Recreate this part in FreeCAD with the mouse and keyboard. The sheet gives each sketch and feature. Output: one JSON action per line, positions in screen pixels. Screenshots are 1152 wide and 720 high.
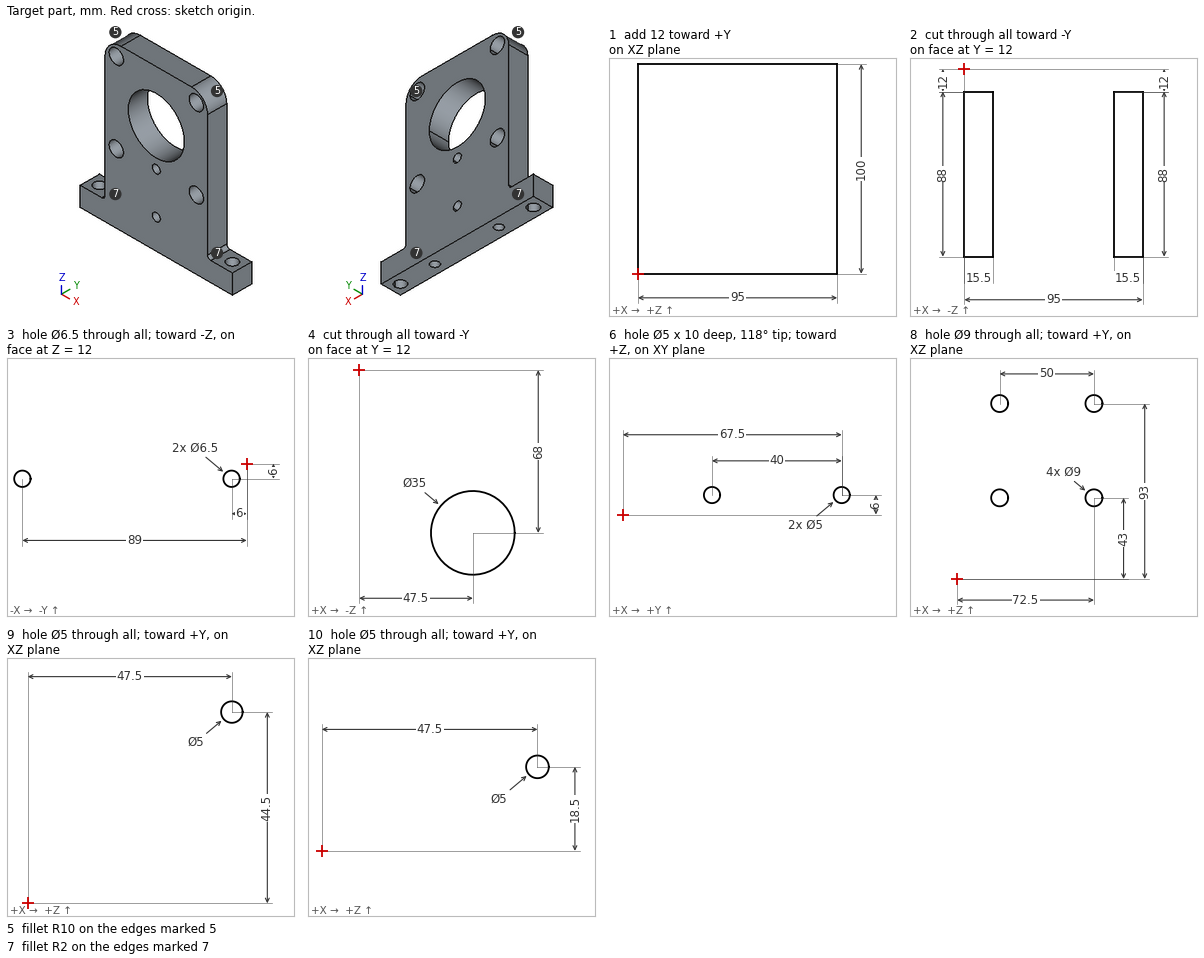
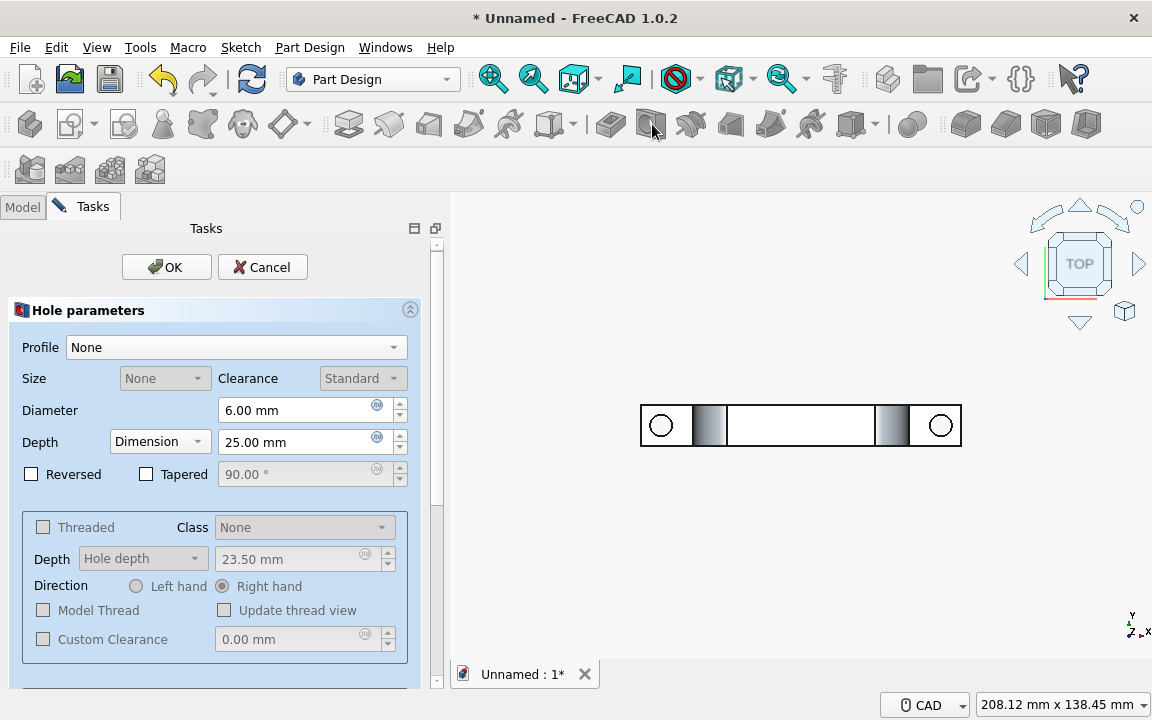
{"action": "triple_click", "coordinate": [305, 410]}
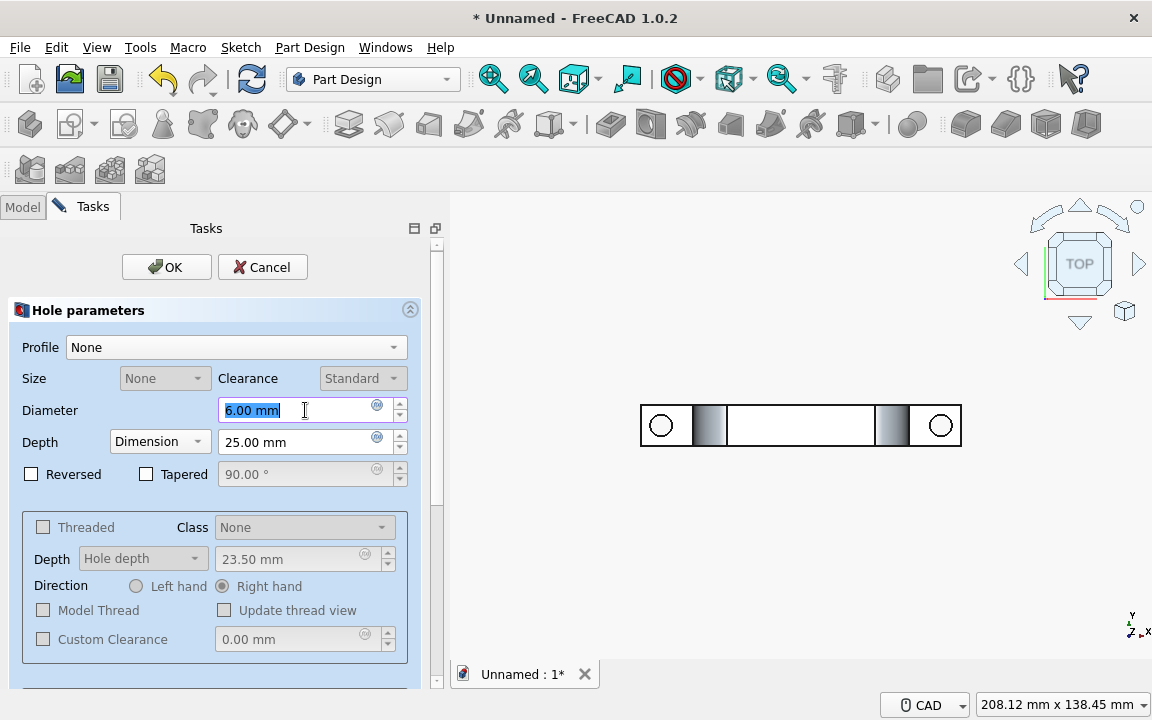
{"action": "type", "text": "5"}
{"action": "key", "text": "Tab"}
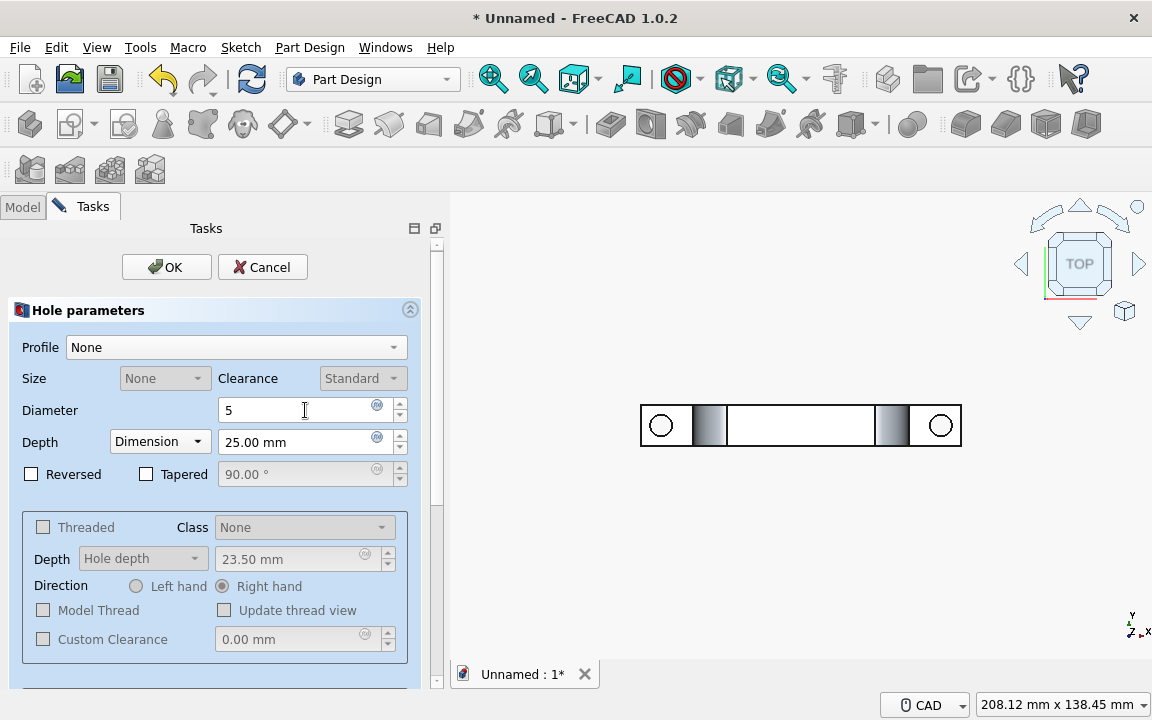
{"action": "triple_click", "coordinate": [305, 442]}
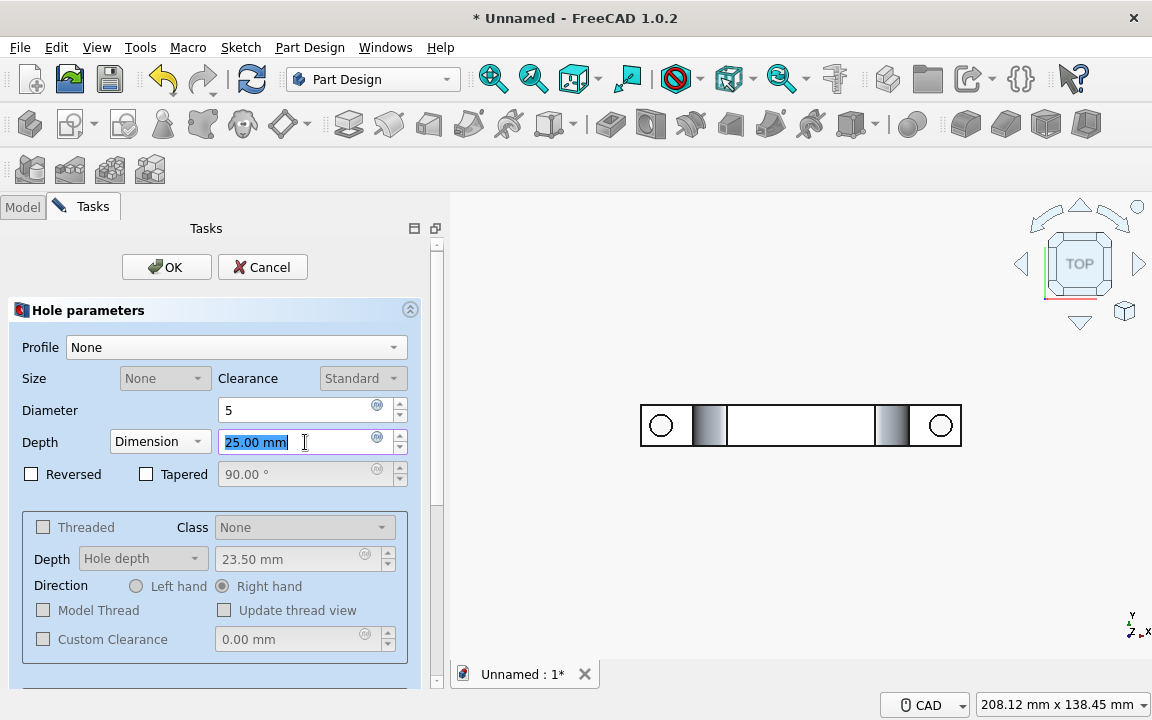
{"action": "type", "text": "10"}
{"action": "key", "text": "Tab"}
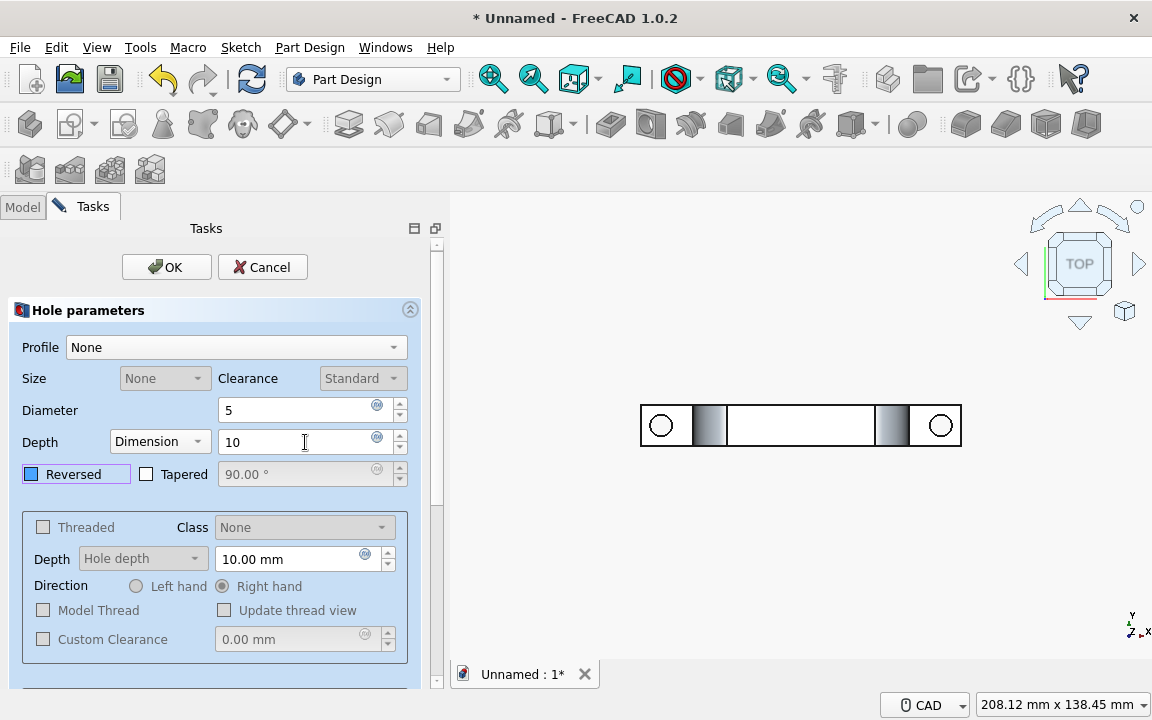
{"action": "left_click", "coordinate": [30, 474]}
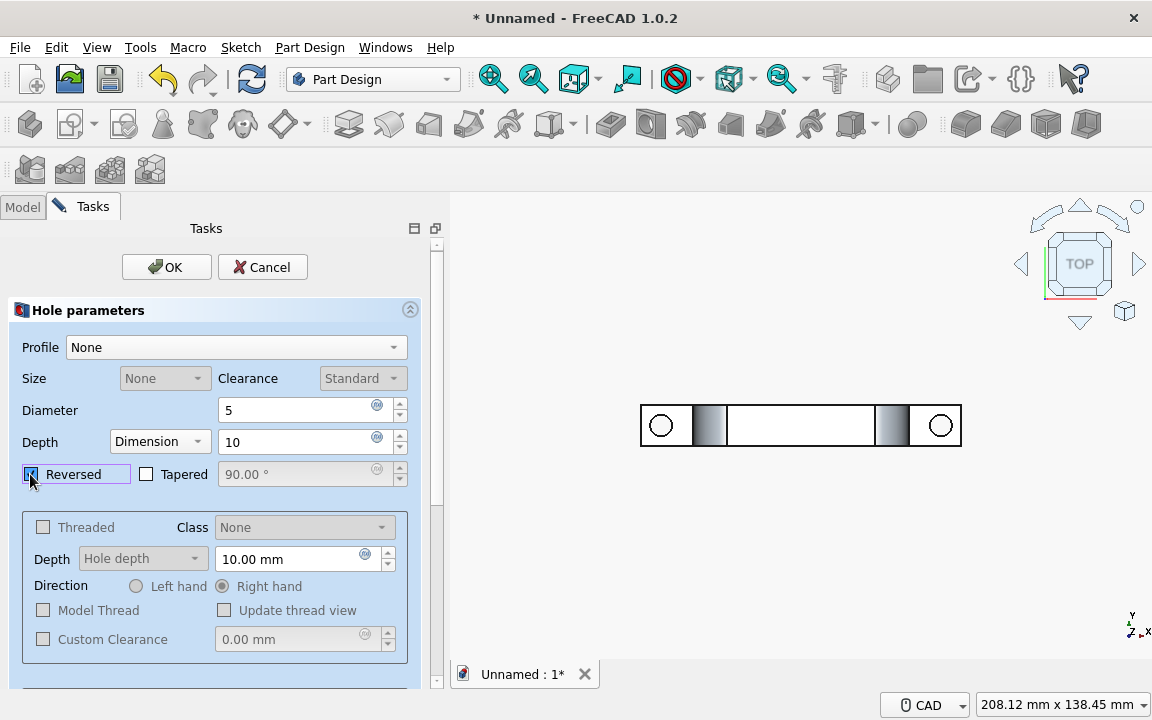
{"action": "left_click", "coordinate": [167, 267]}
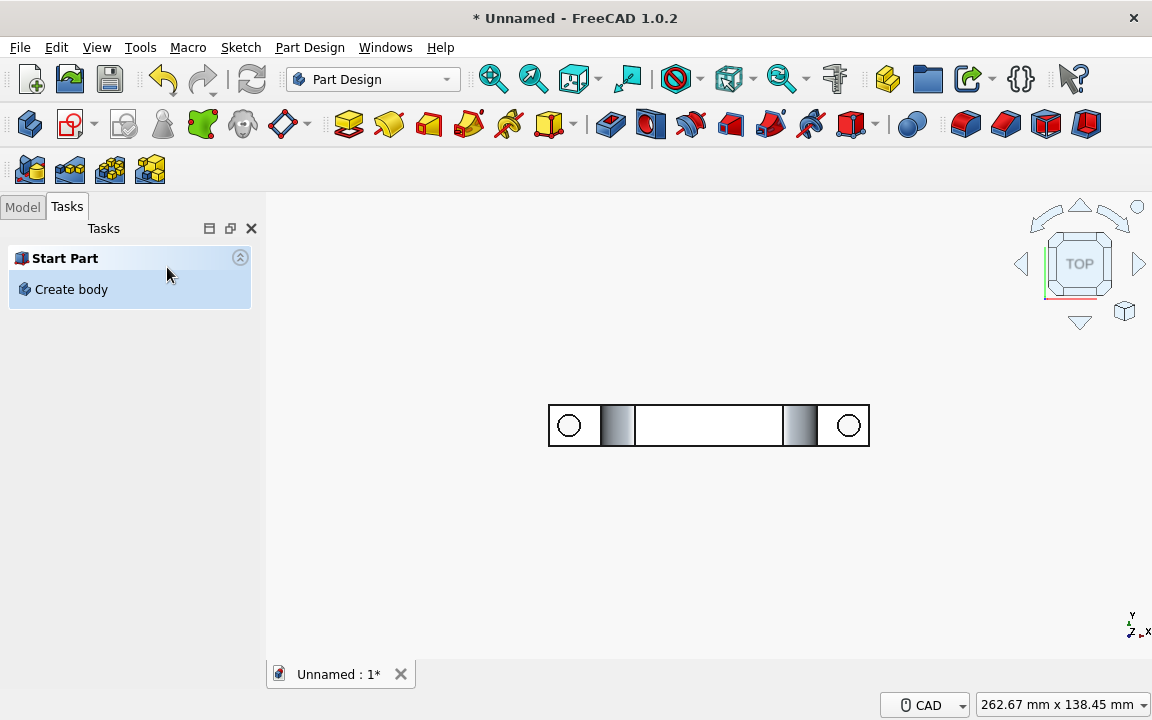
{"action": "left_click", "coordinate": [494, 80]}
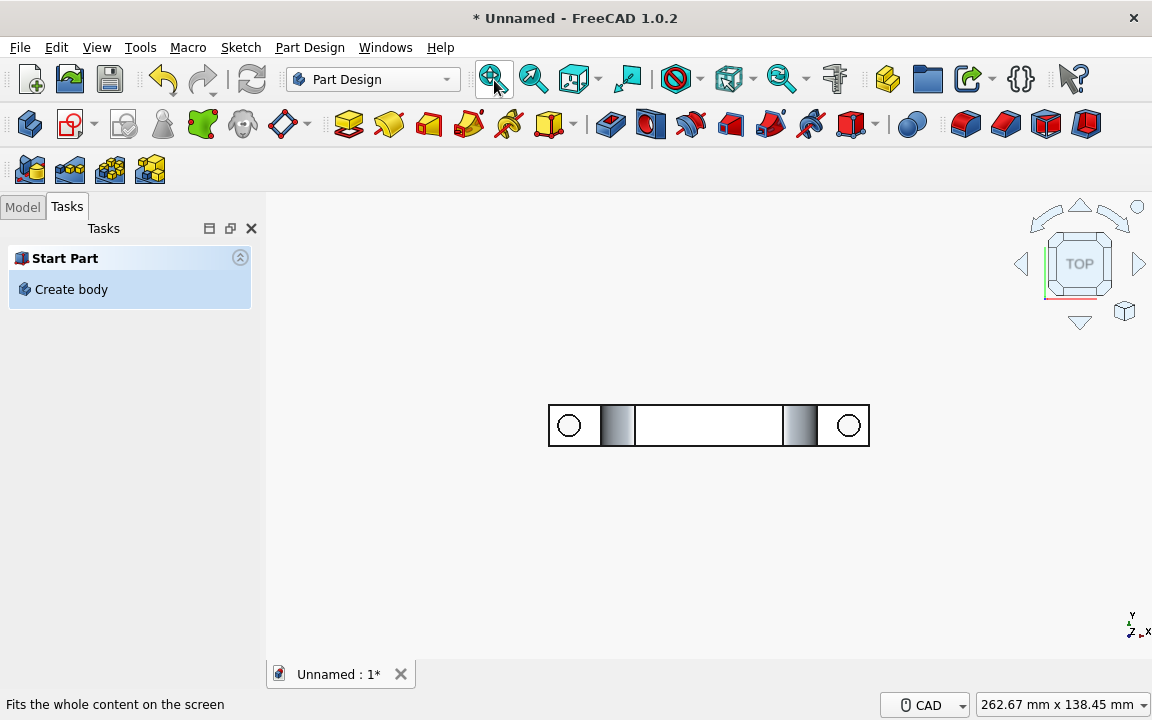
{"action": "key", "text": "0"}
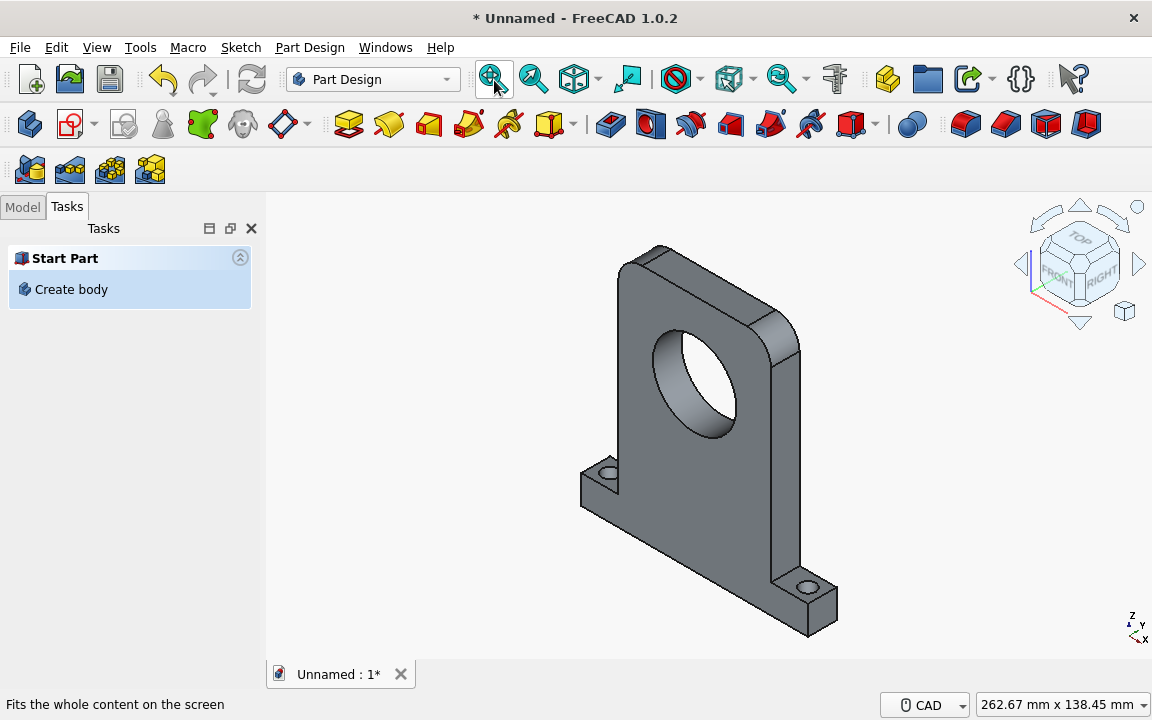
{"action": "key", "text": "2"}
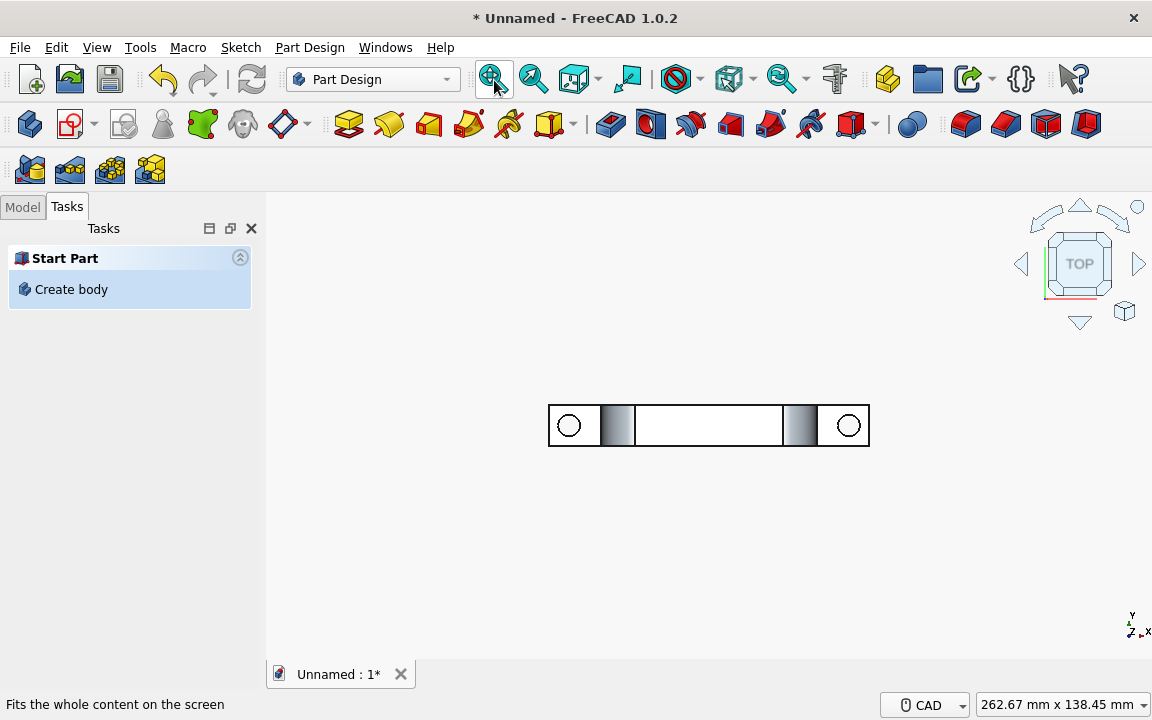
{"action": "left_click", "coordinate": [494, 80]}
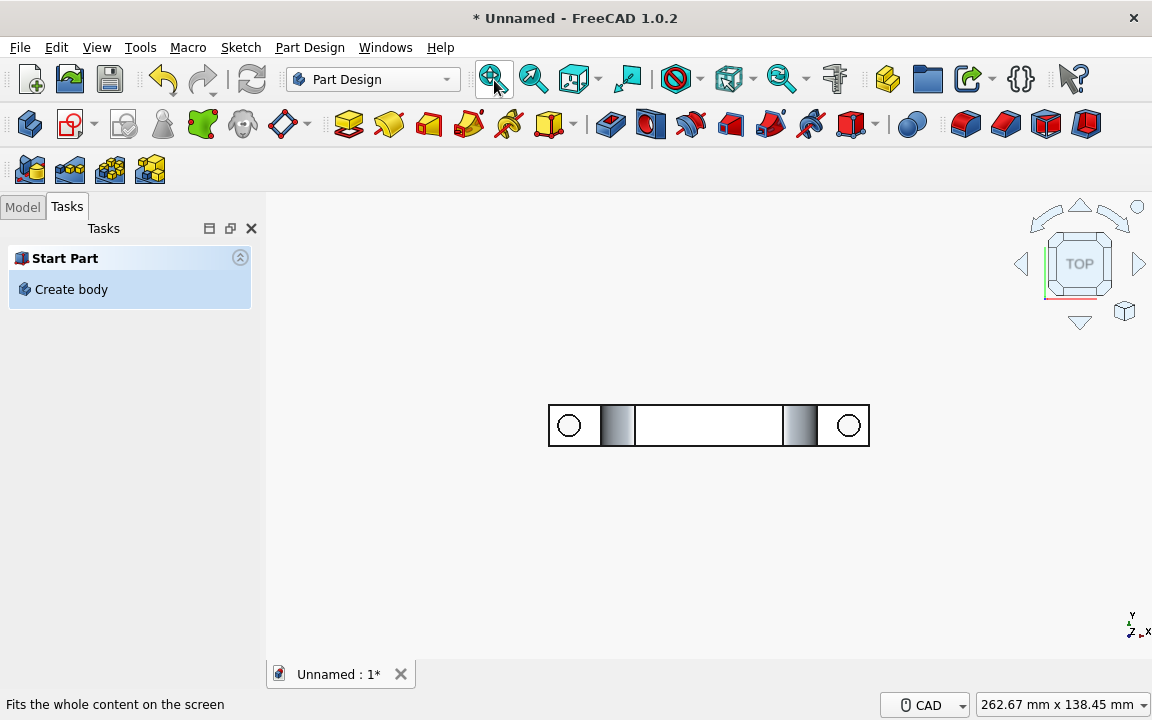
{"action": "key", "text": "1"}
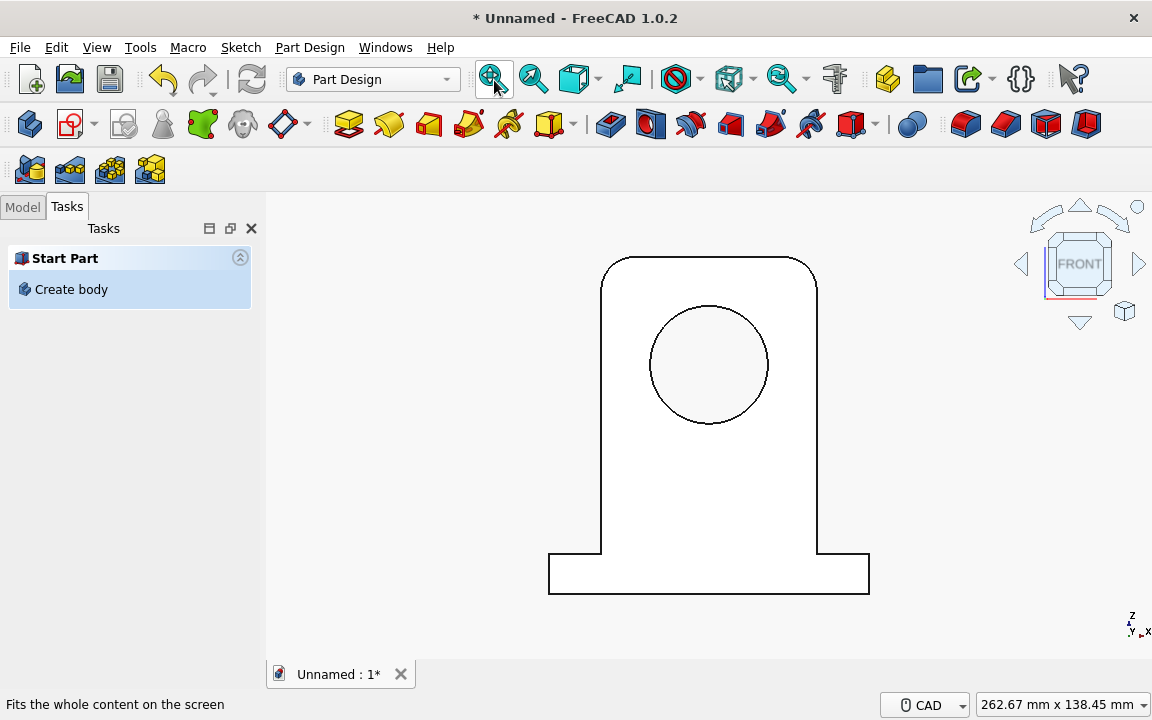
{"action": "key", "text": "3"}